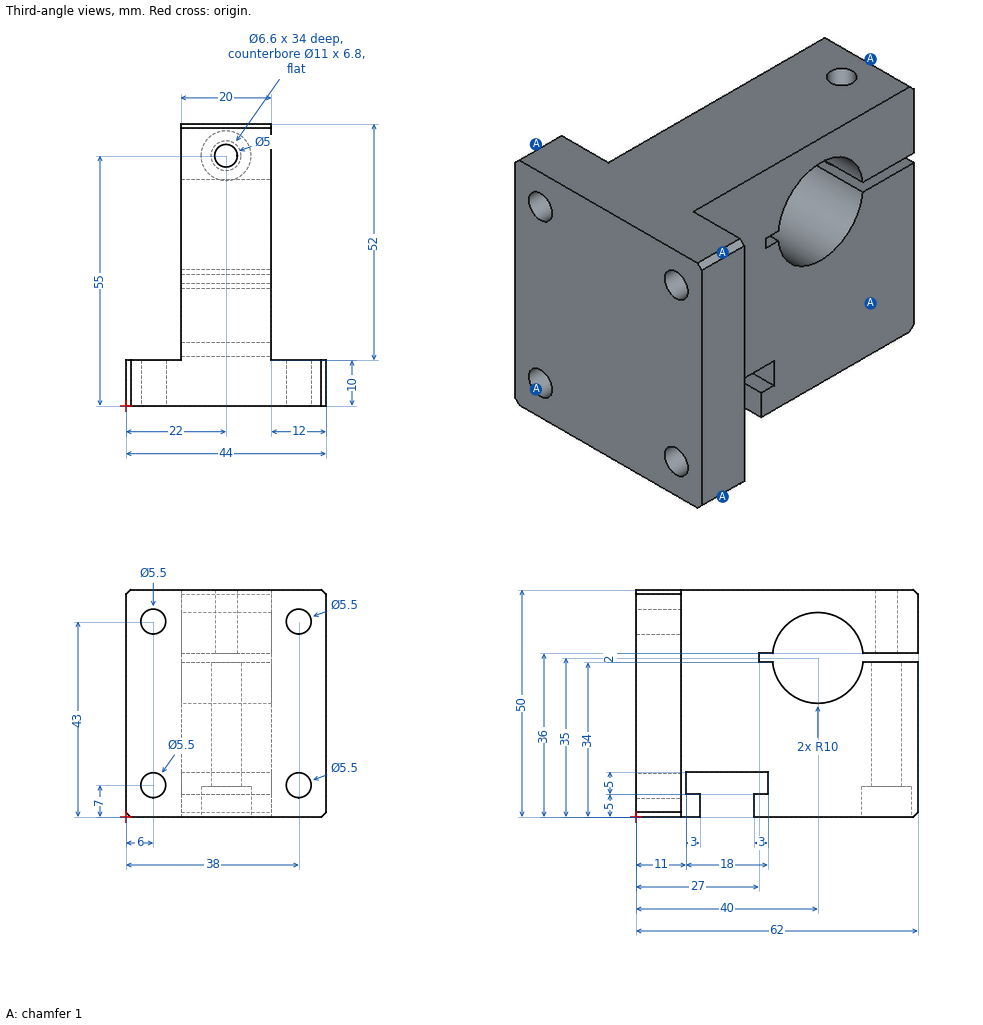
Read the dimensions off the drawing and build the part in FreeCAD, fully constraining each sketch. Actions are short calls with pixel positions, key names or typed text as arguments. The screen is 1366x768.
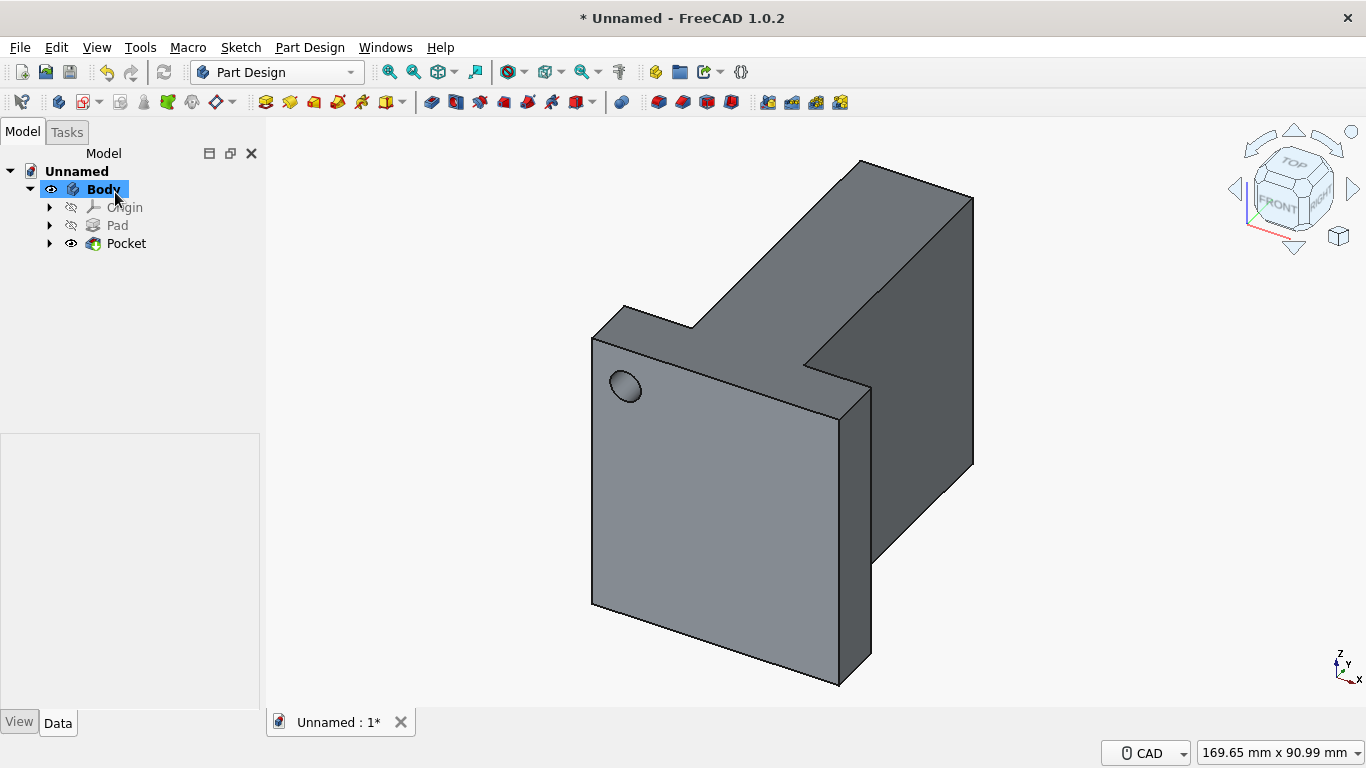
click(715, 511)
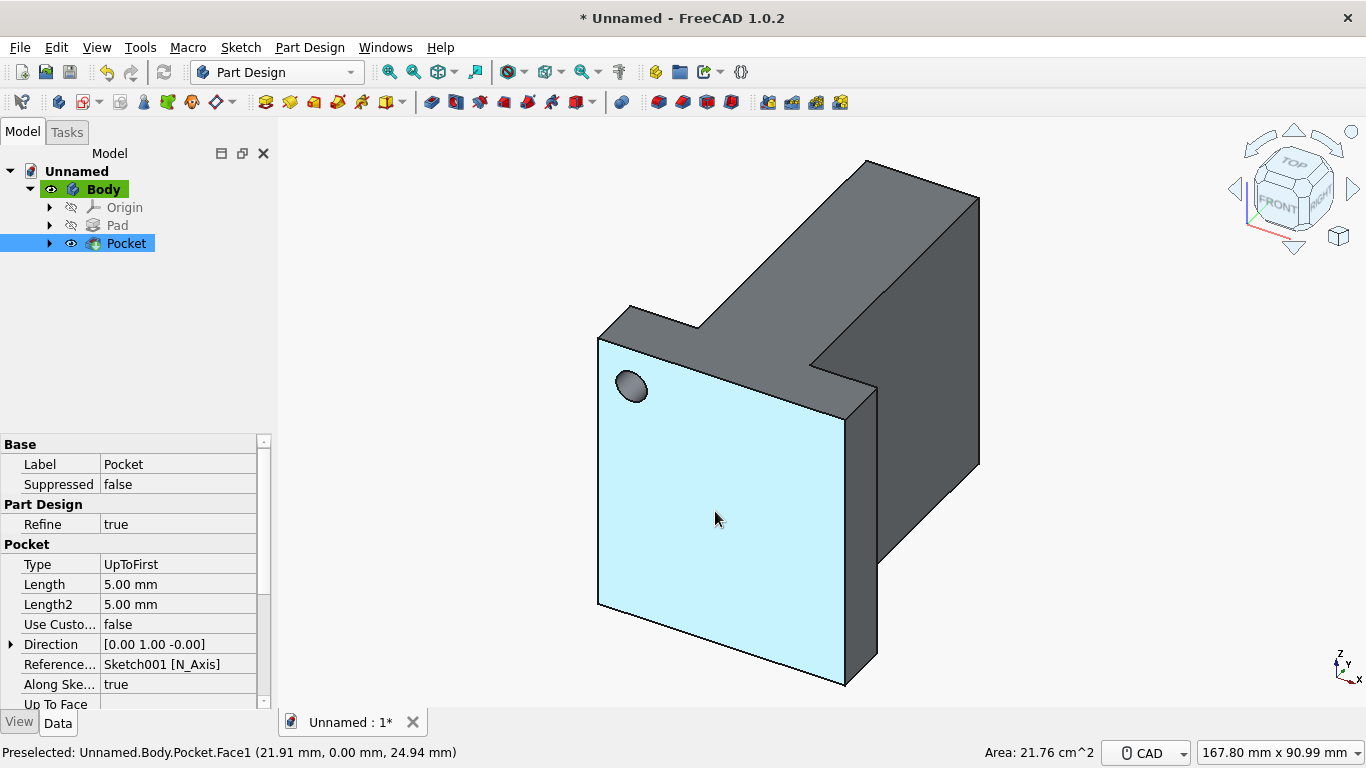
click(84, 102)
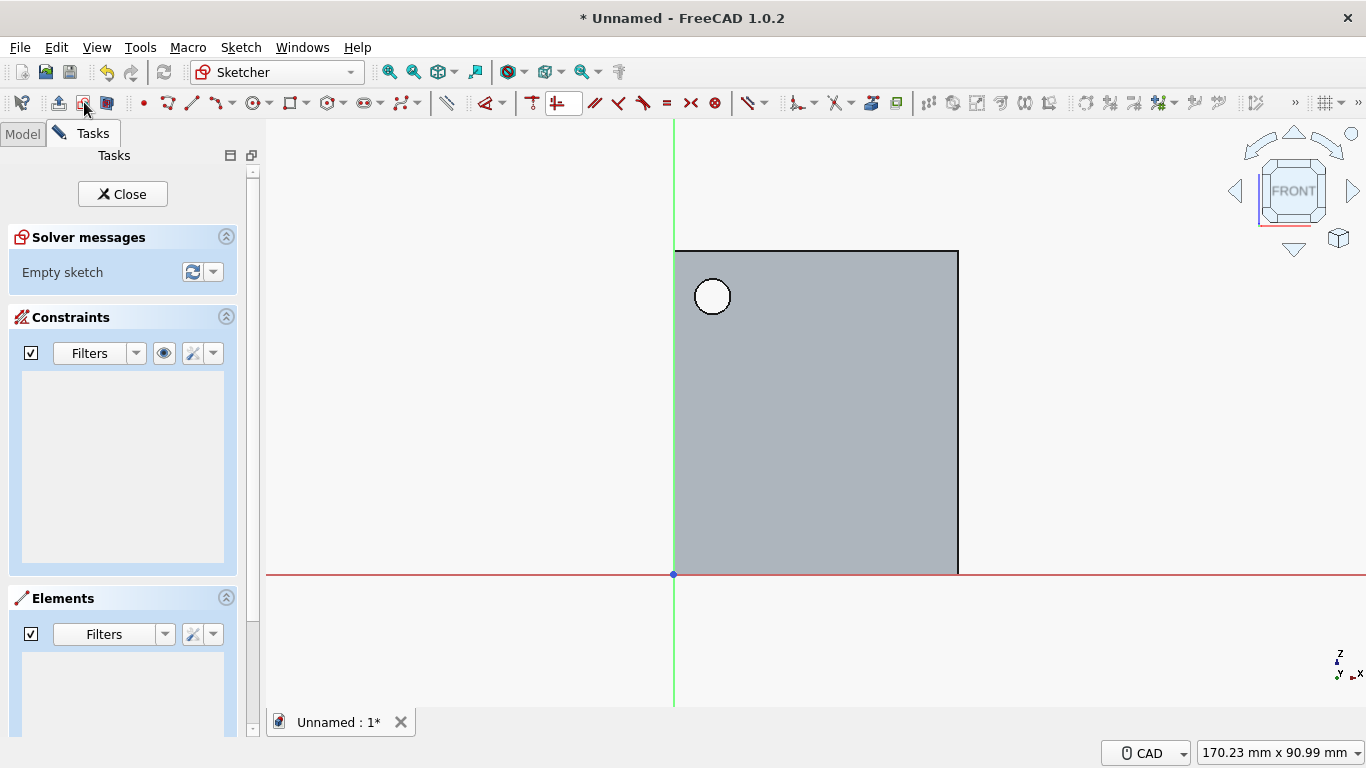
scroll(693, 569, up, 9)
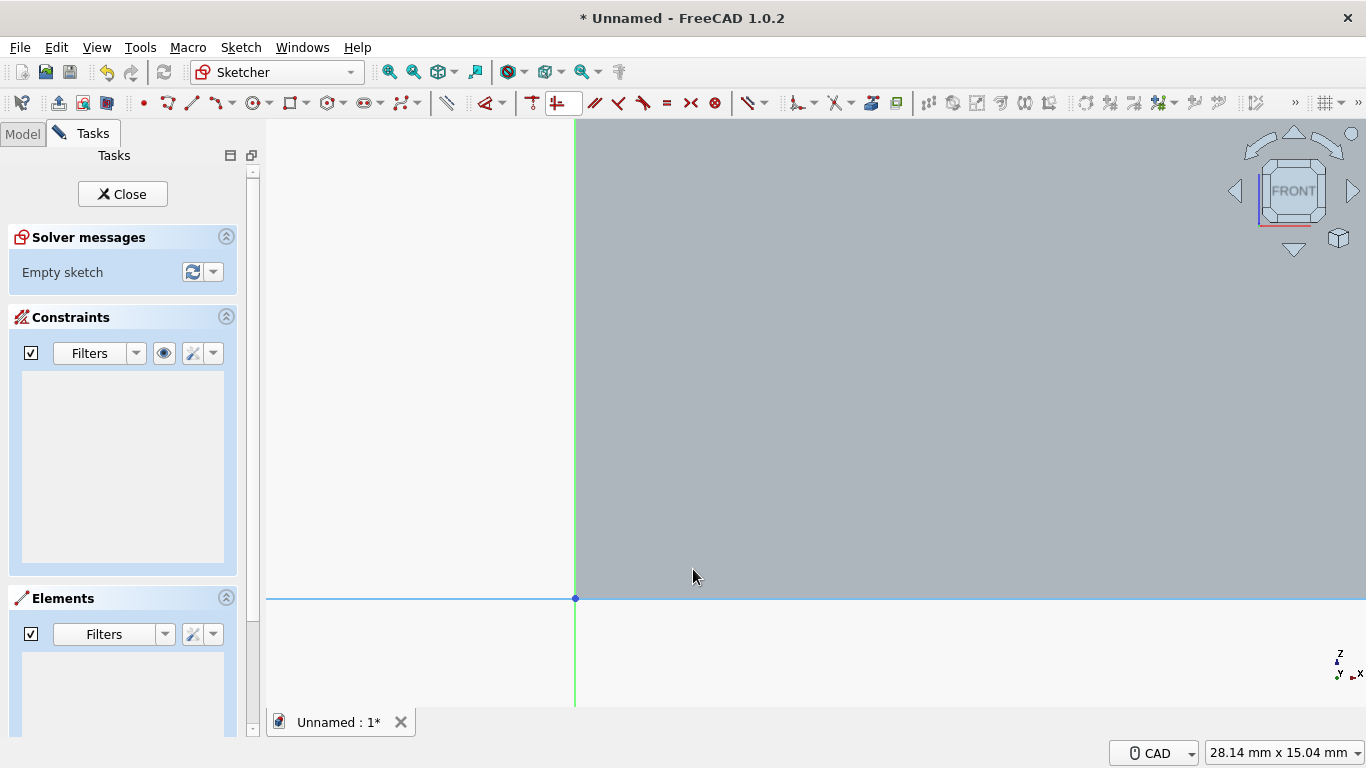
click(254, 104)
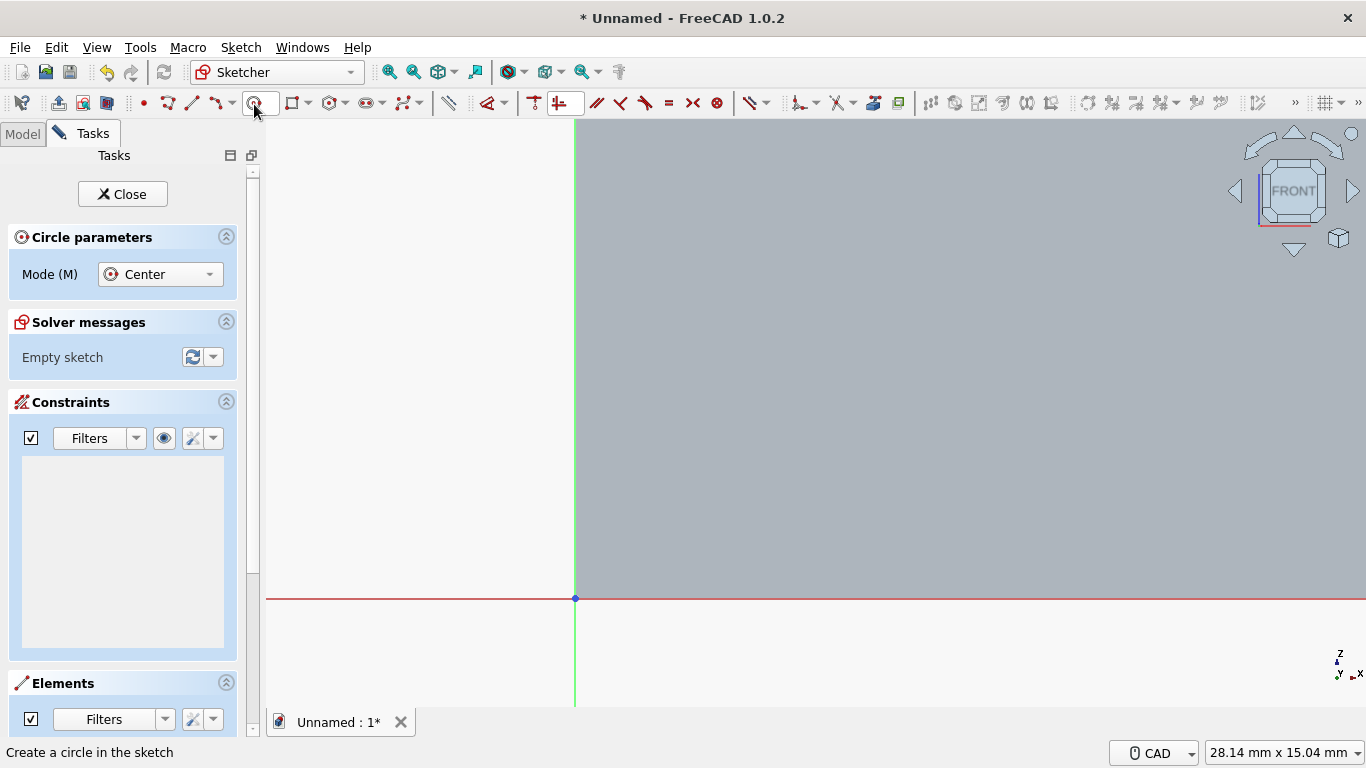
click(810, 325)
move(886, 249)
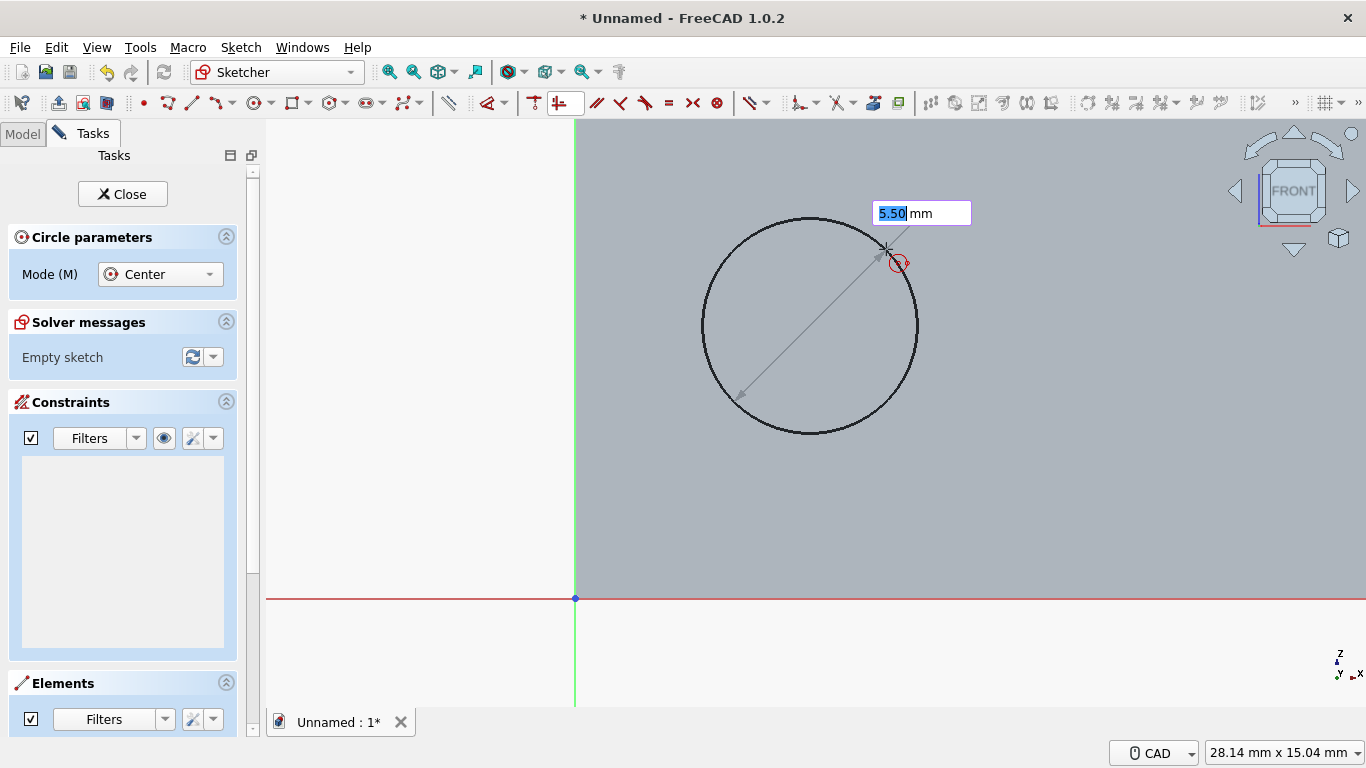
text(5.5)
key(Return)
key(Escape)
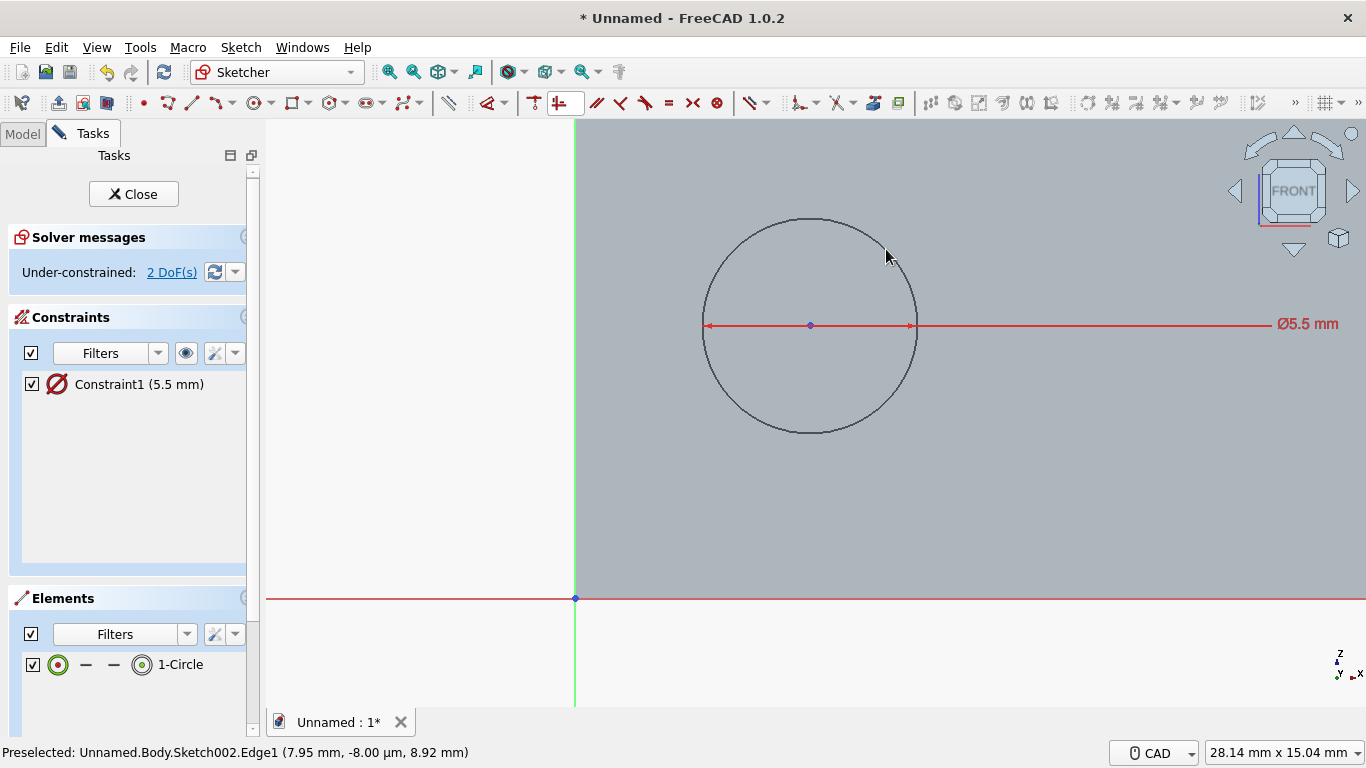
click(488, 104)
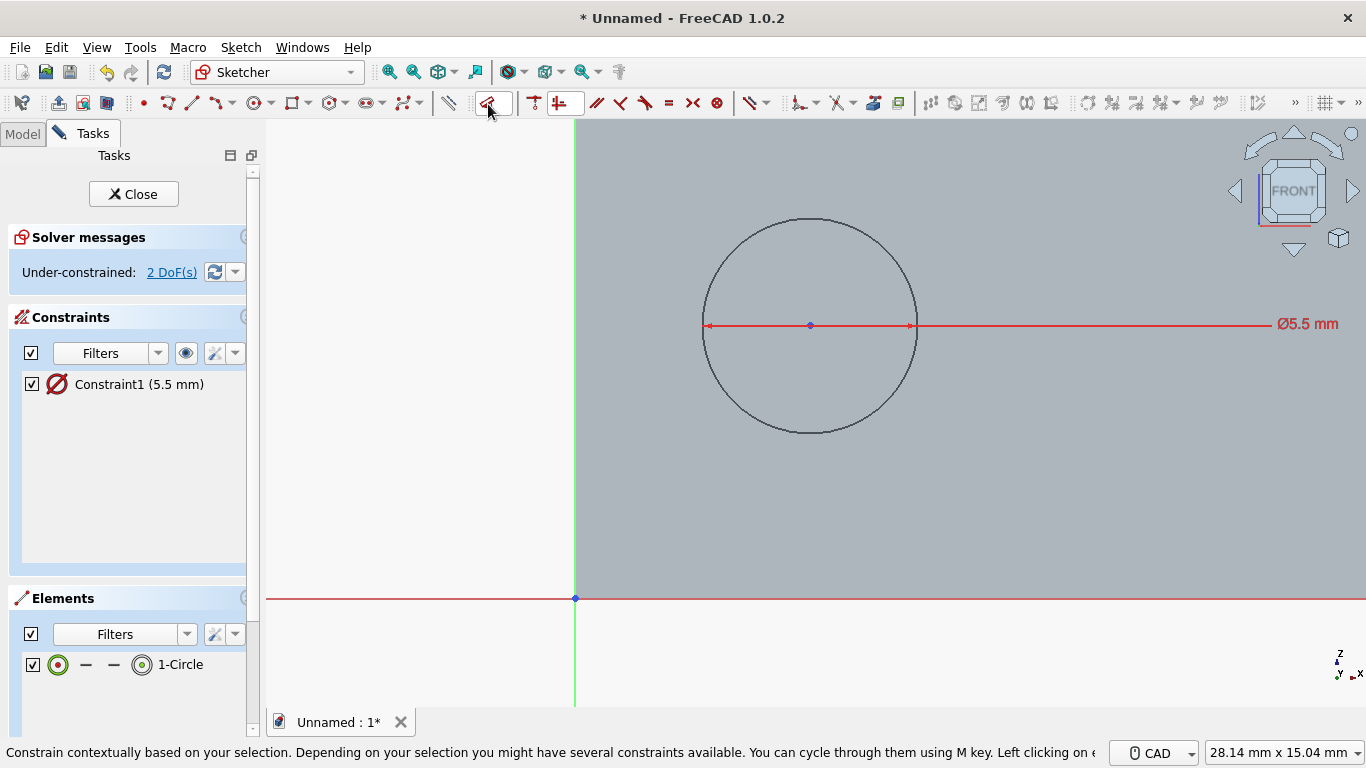
click(810, 326)
click(693, 633)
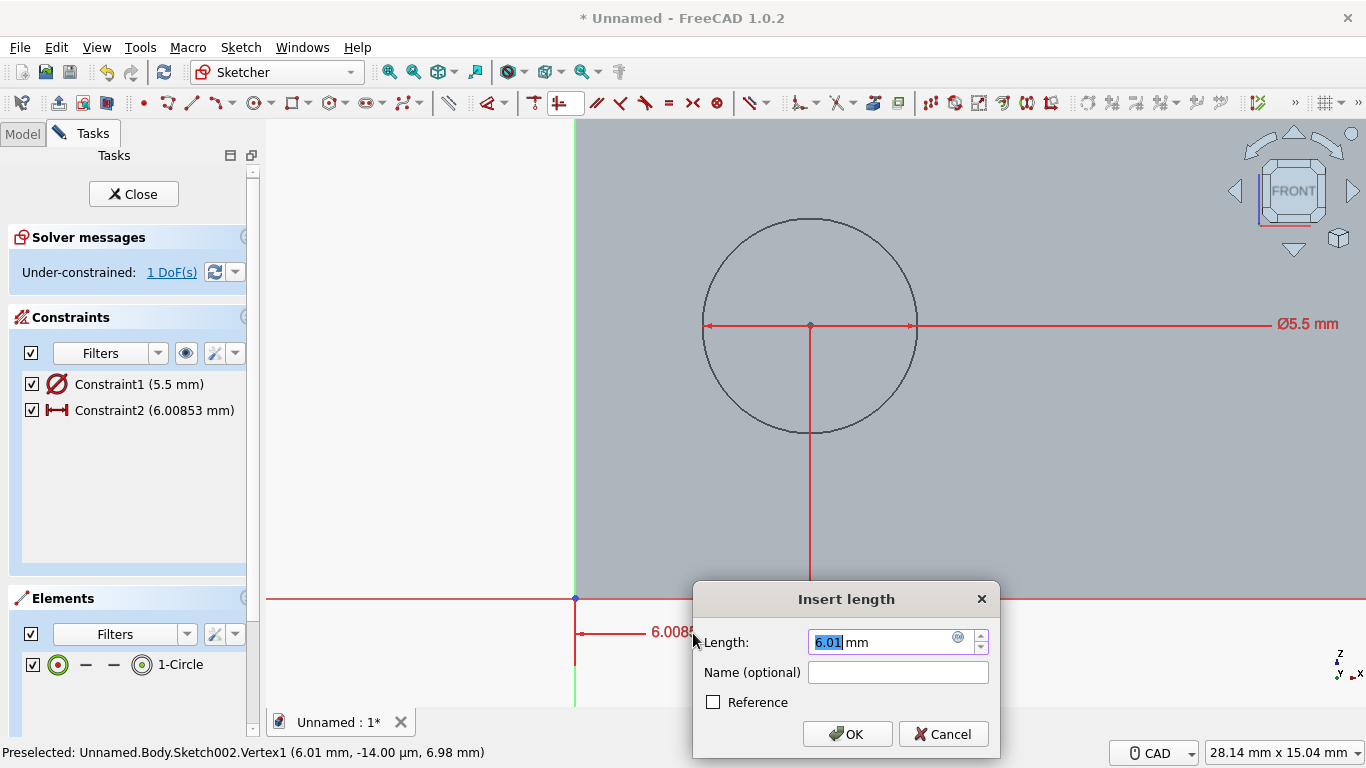
text(6)
key(Return)